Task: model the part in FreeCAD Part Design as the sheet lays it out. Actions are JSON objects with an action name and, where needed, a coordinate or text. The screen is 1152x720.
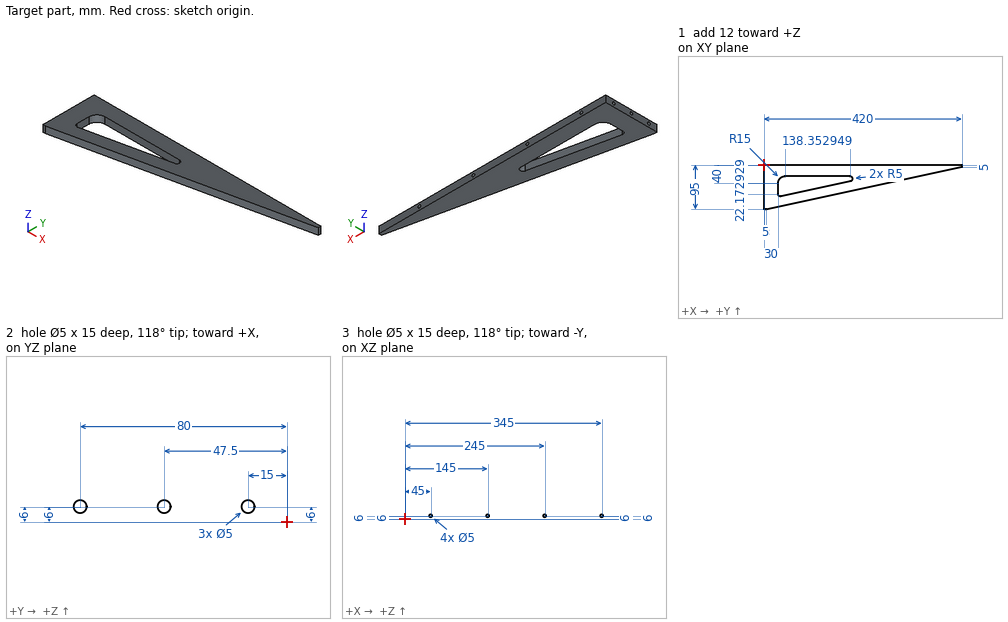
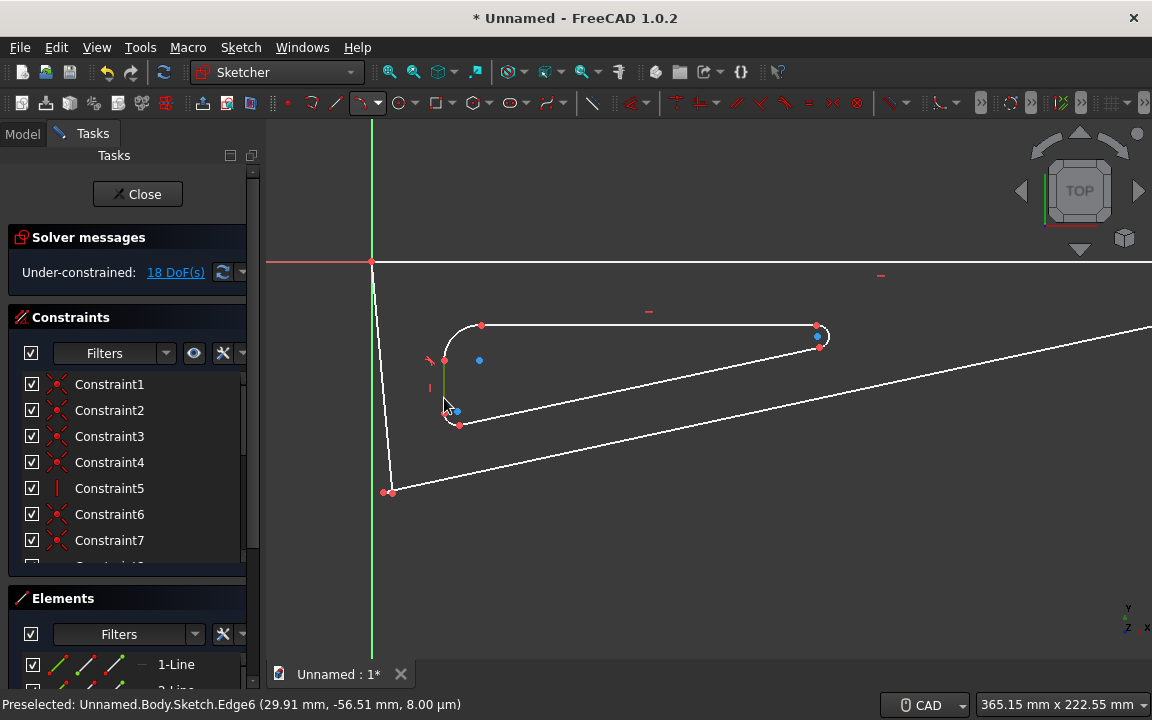
{"action": "scroll", "coordinate": [450, 423], "scroll_direction": "up", "scroll_amount": 2}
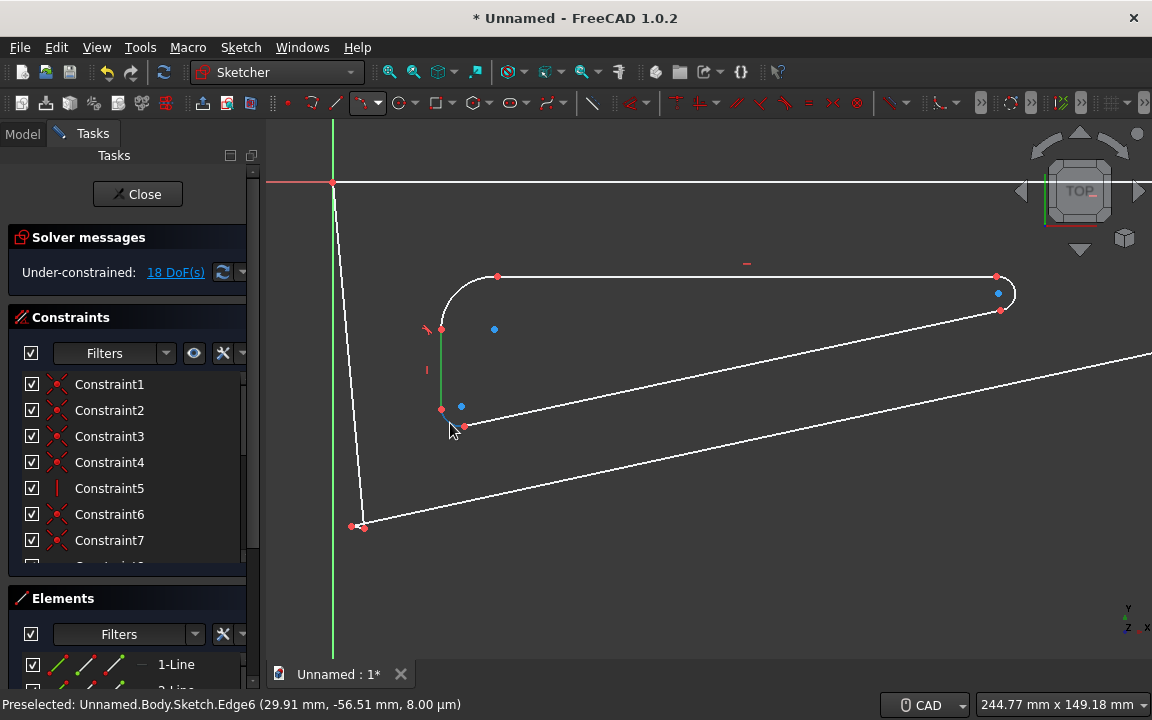
{"action": "left_click", "coordinate": [449, 422]}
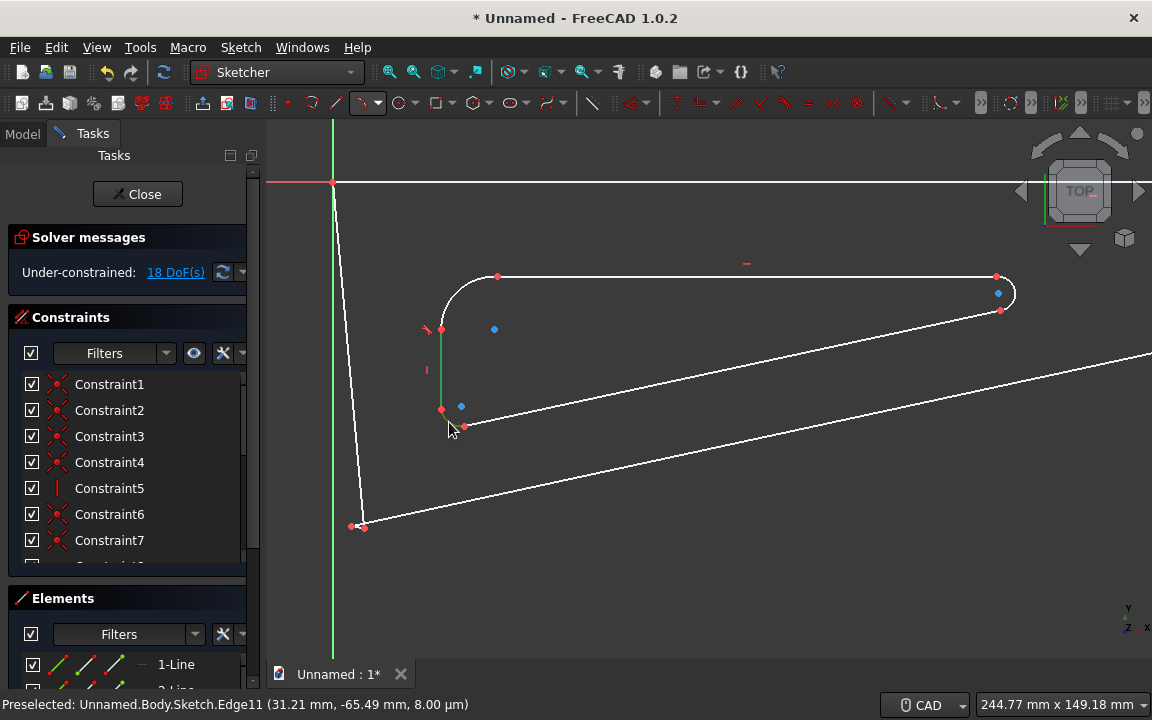
{"action": "left_click", "coordinate": [786, 104]}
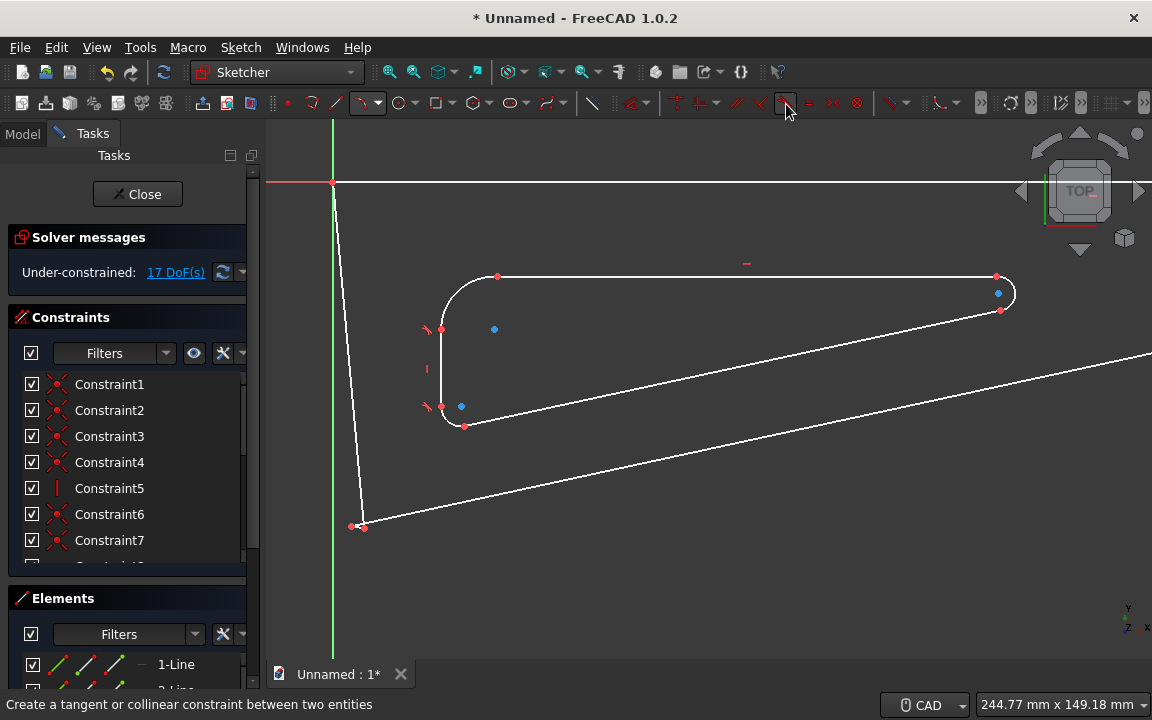
{"action": "left_click", "coordinate": [647, 277]}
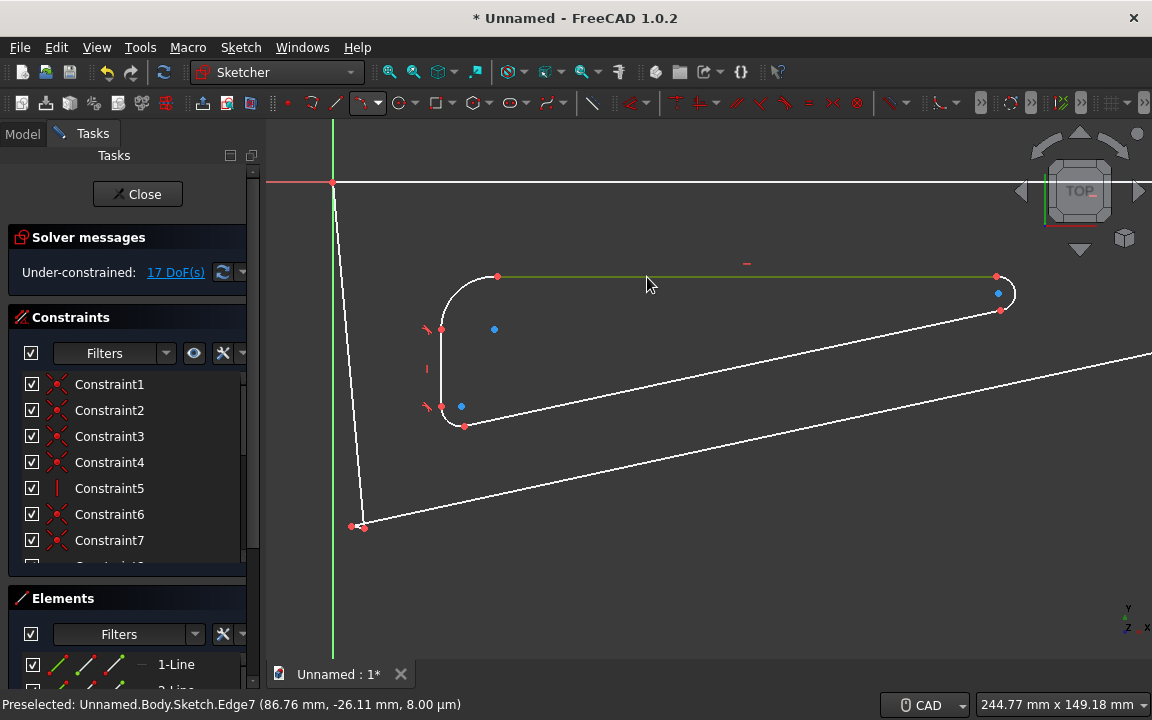
{"action": "left_click", "coordinate": [472, 282]}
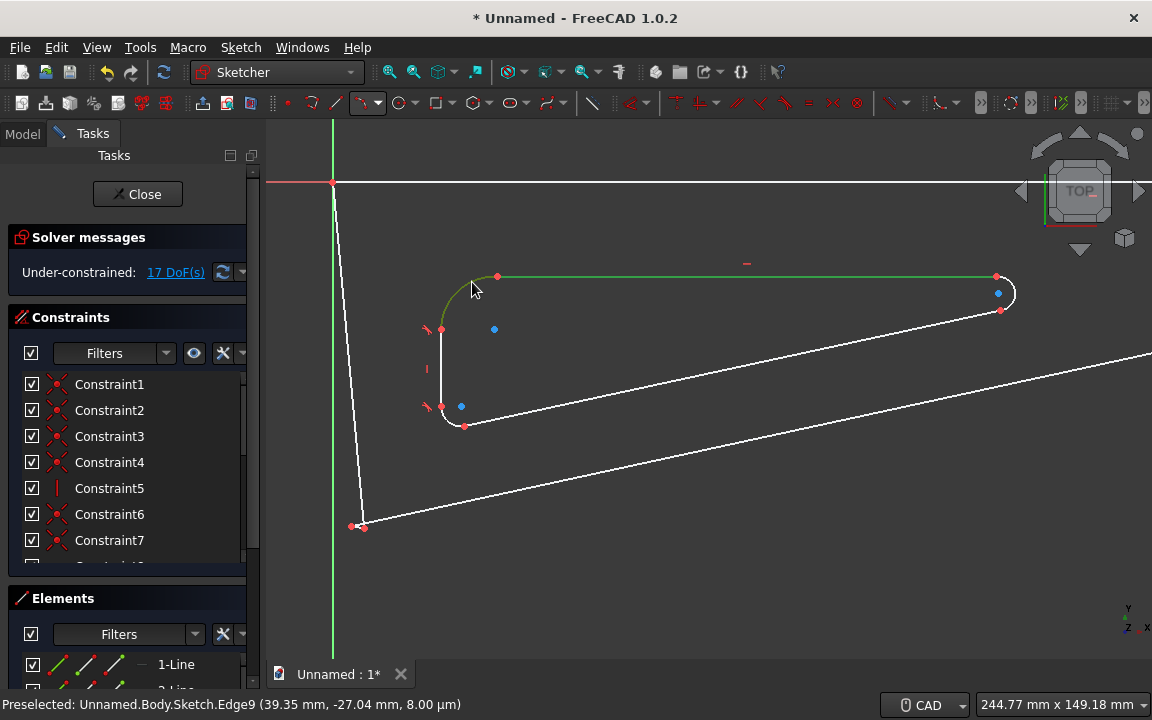
{"action": "left_click", "coordinate": [786, 104]}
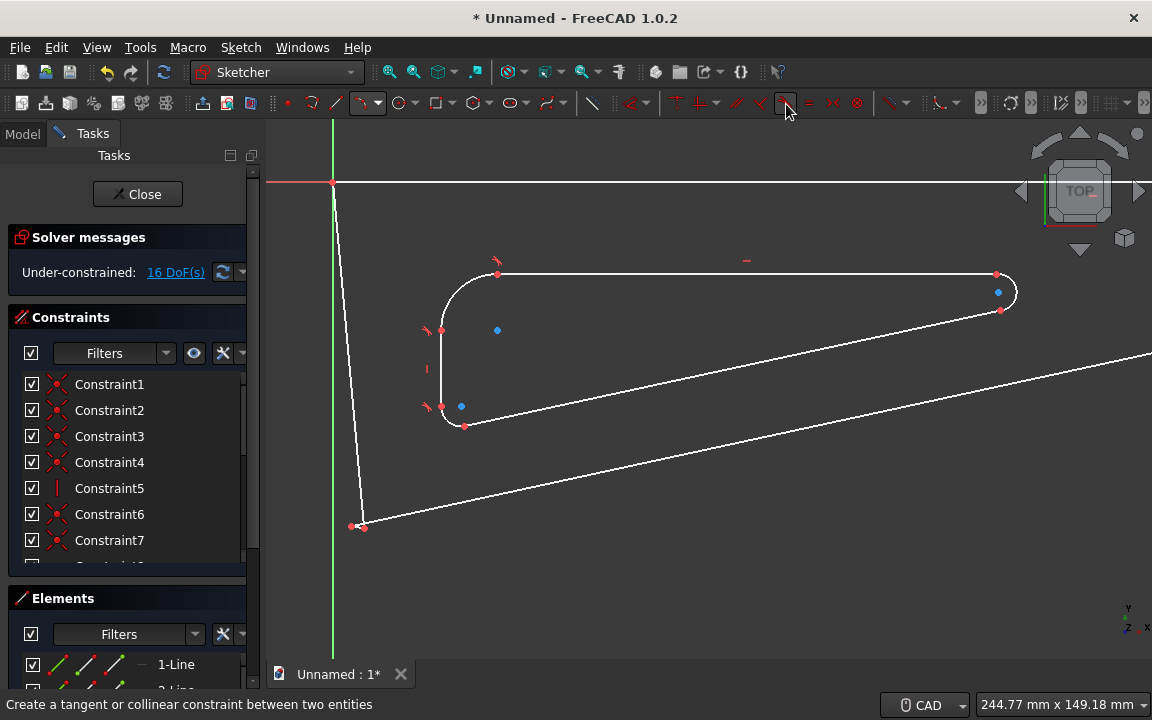
{"action": "left_click", "coordinate": [647, 274]}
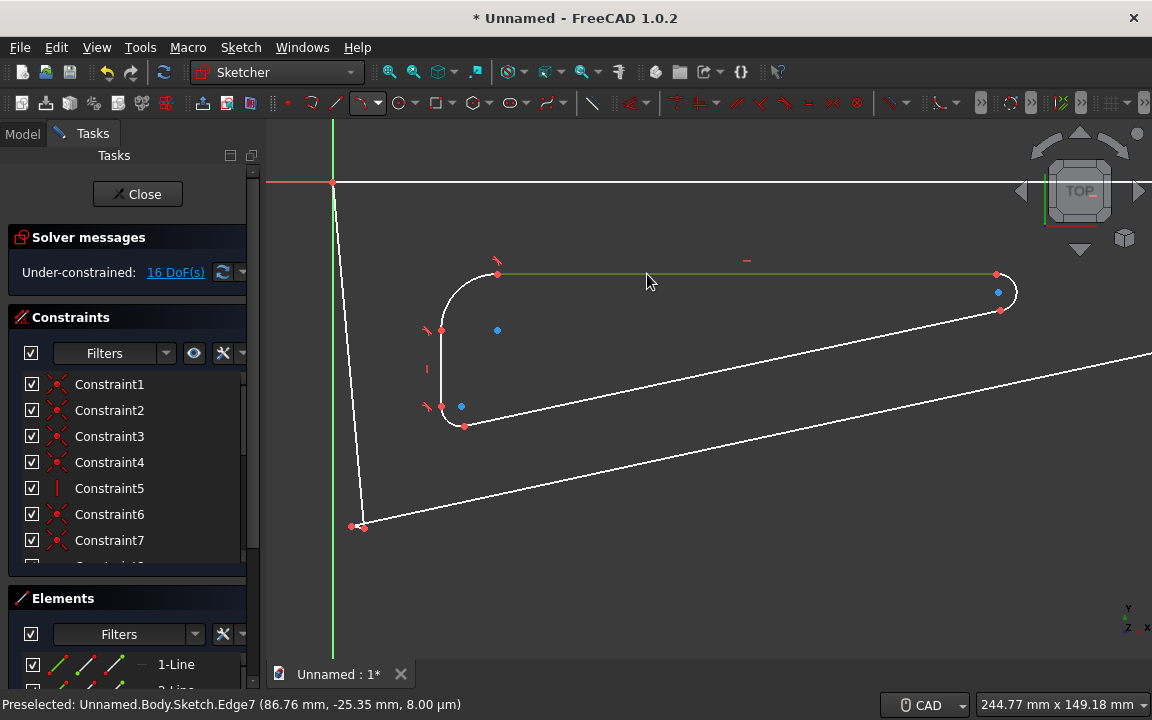
{"action": "scroll", "coordinate": [445, 404], "scroll_direction": "down", "scroll_amount": 6}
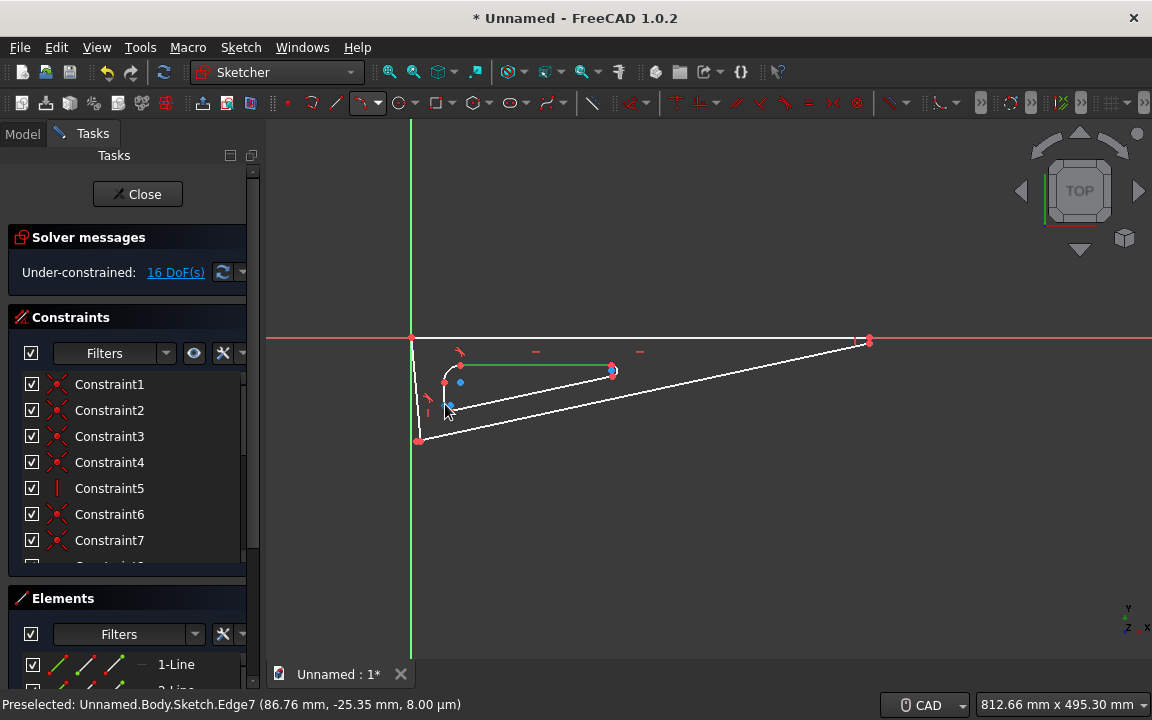
{"action": "scroll", "coordinate": [617, 373], "scroll_direction": "up", "scroll_amount": 6}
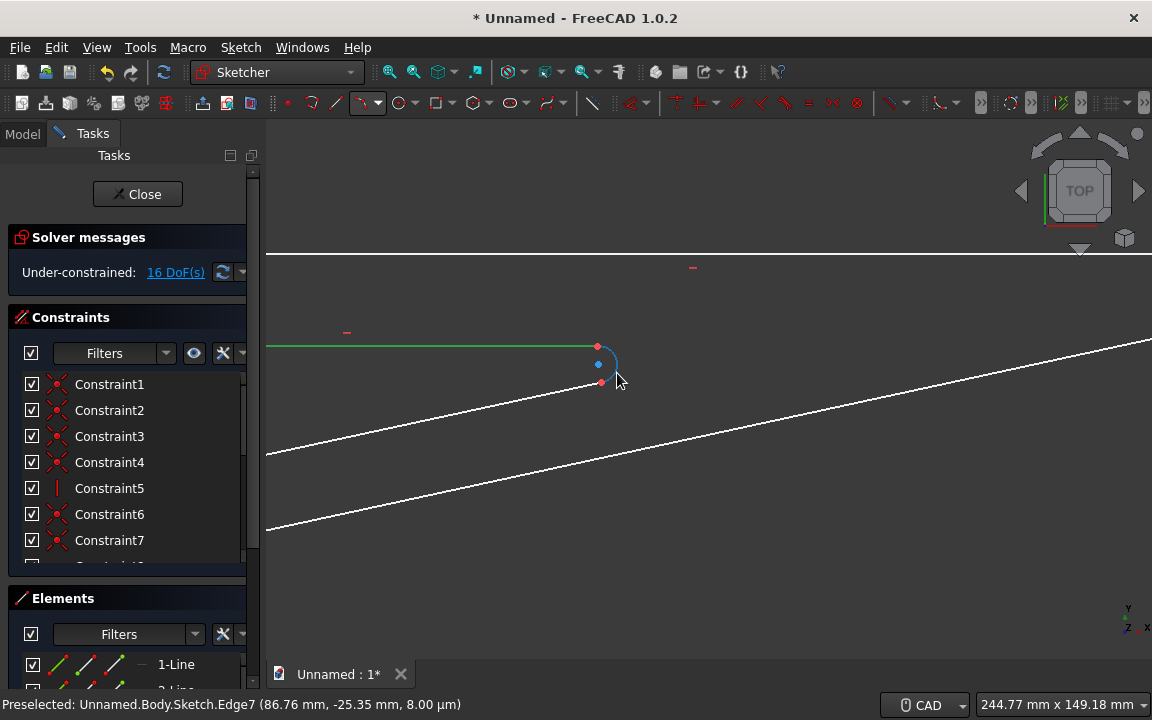
{"action": "left_click", "coordinate": [615, 373]}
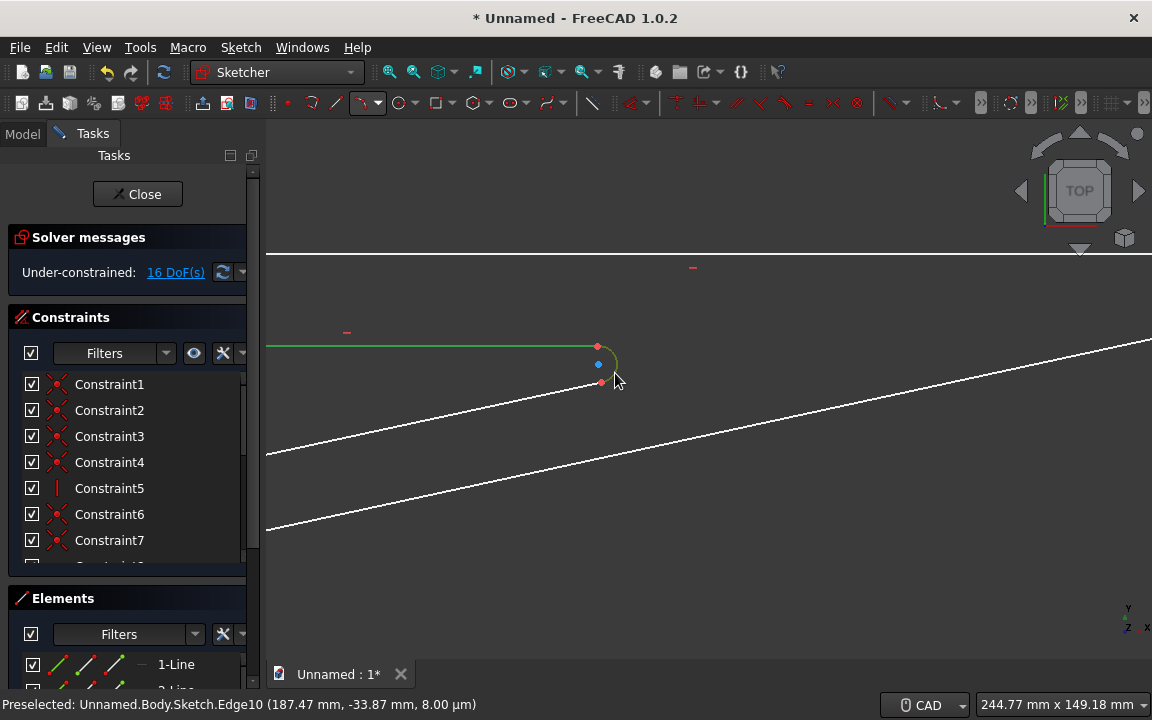
{"action": "left_click", "coordinate": [786, 104]}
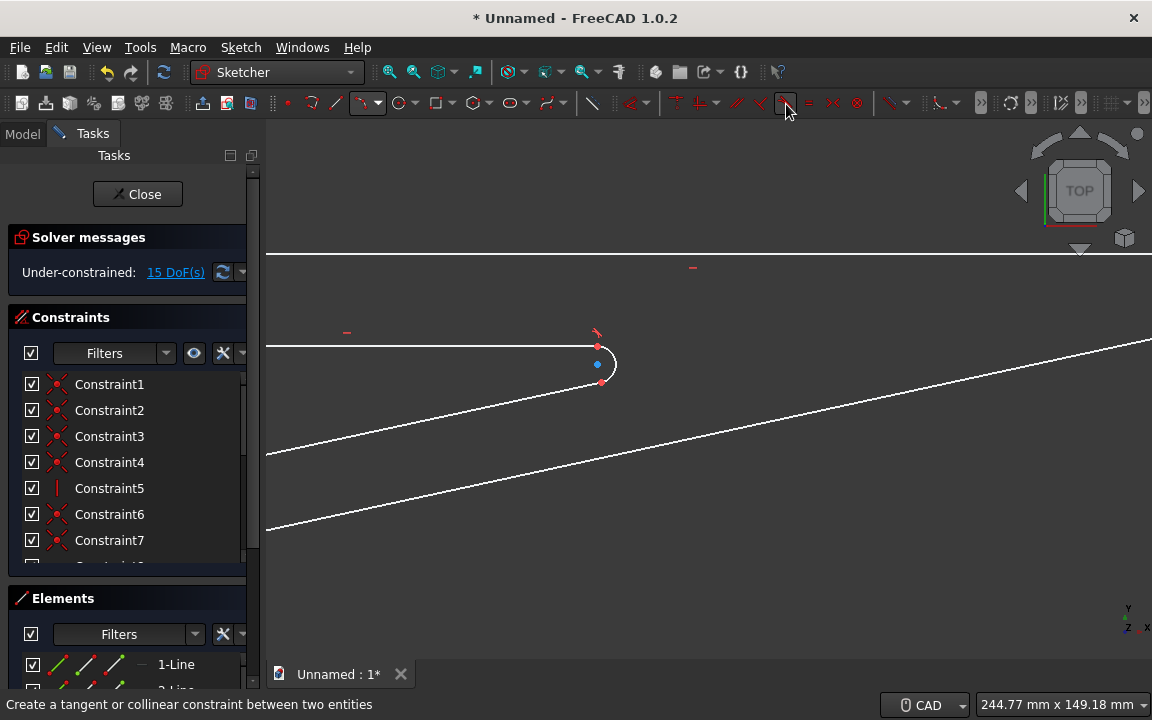
{"action": "left_click", "coordinate": [440, 417]}